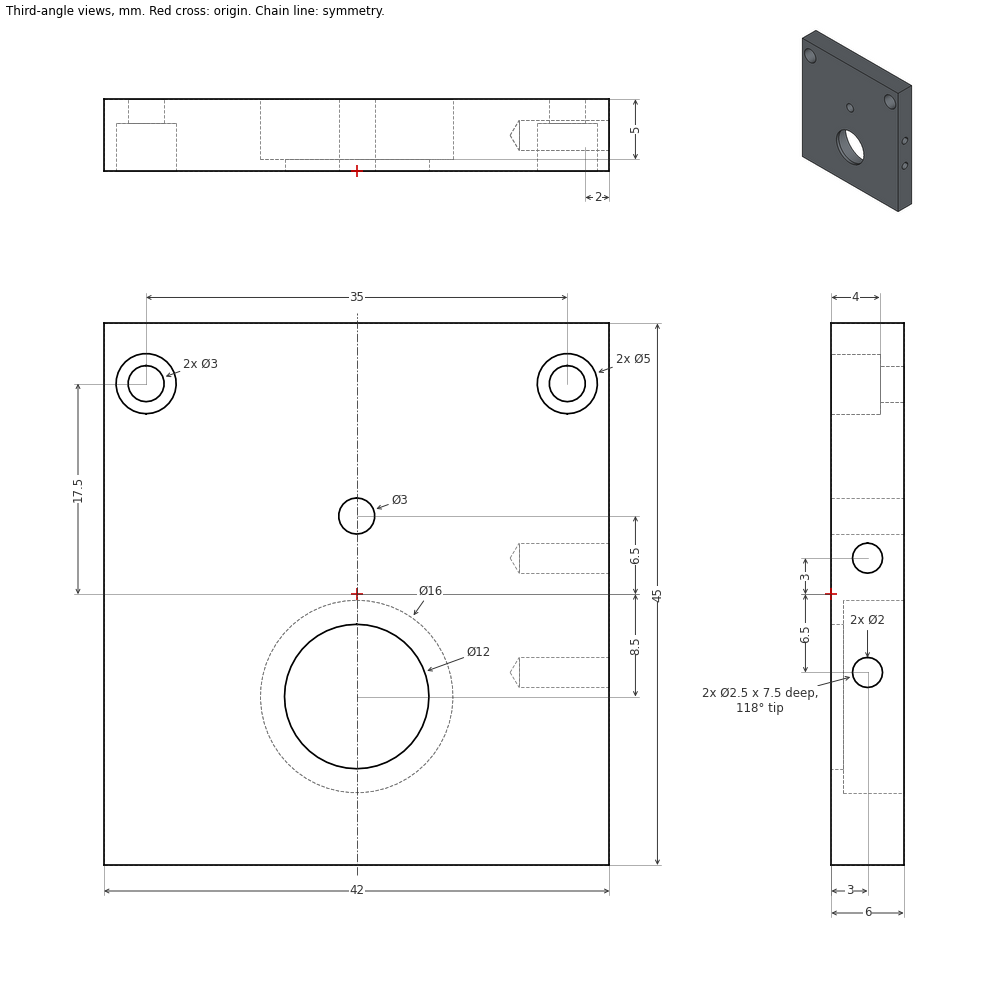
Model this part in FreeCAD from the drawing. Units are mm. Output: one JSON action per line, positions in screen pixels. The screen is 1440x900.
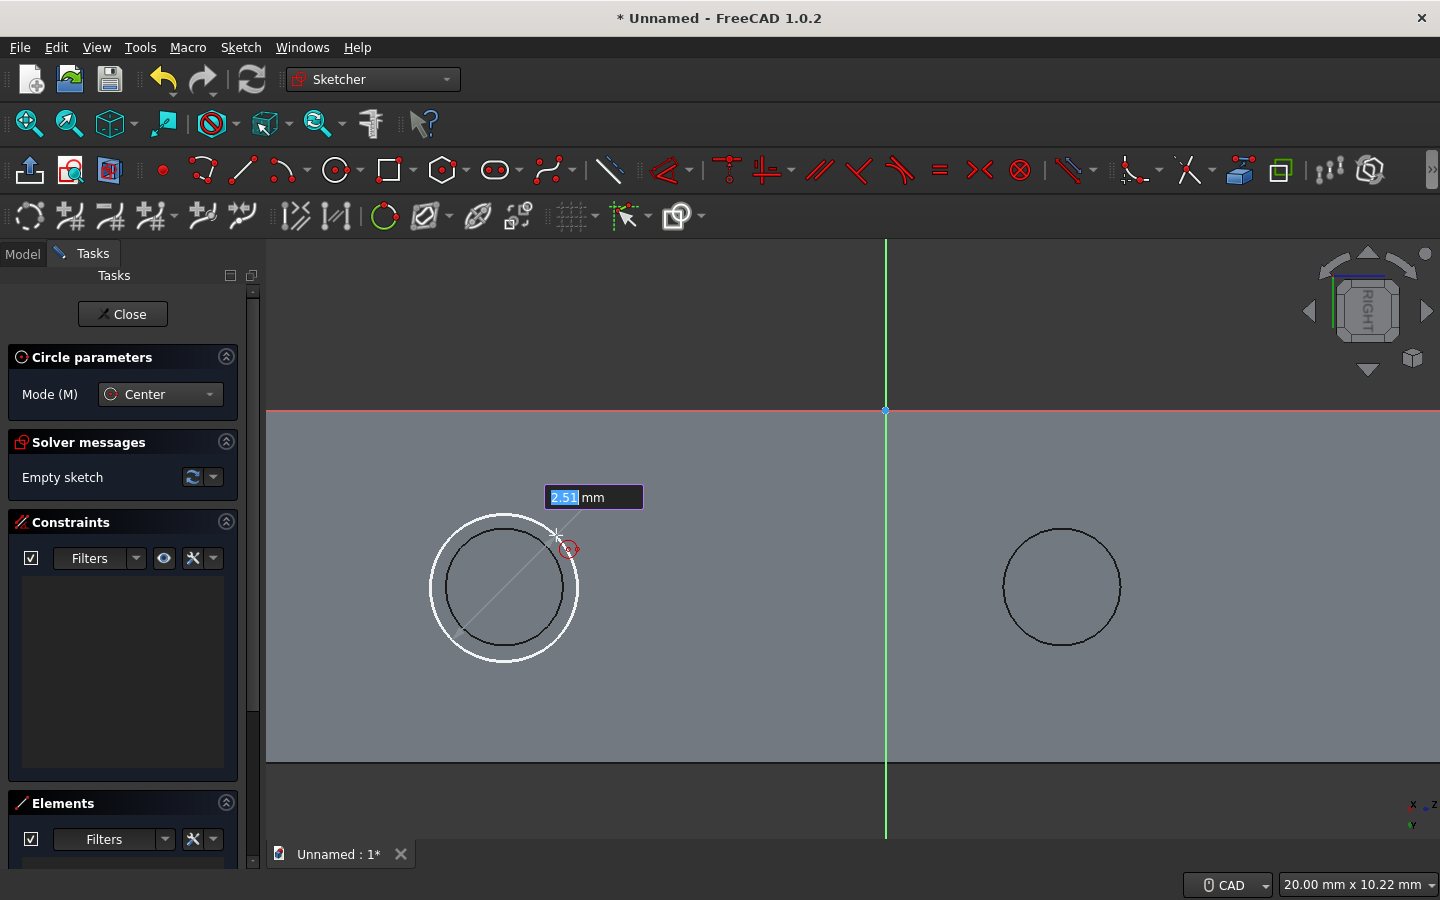
{"action": "type", "text": "2.5"}
{"action": "key", "text": "Return"}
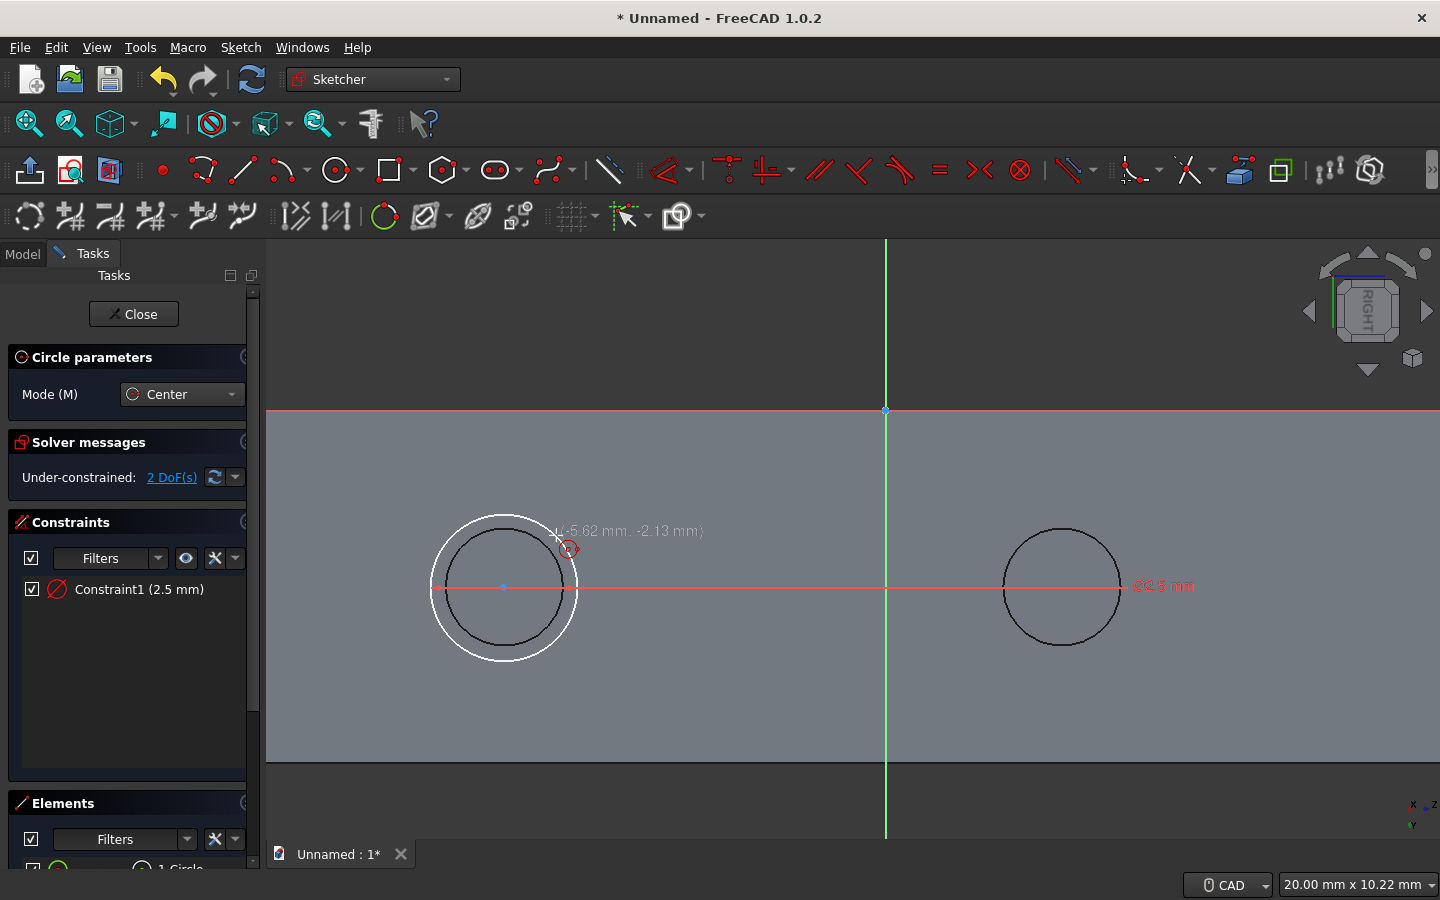
{"action": "left_click", "coordinate": [1062, 587]}
{"action": "mouse_move", "coordinate": [1114, 535]}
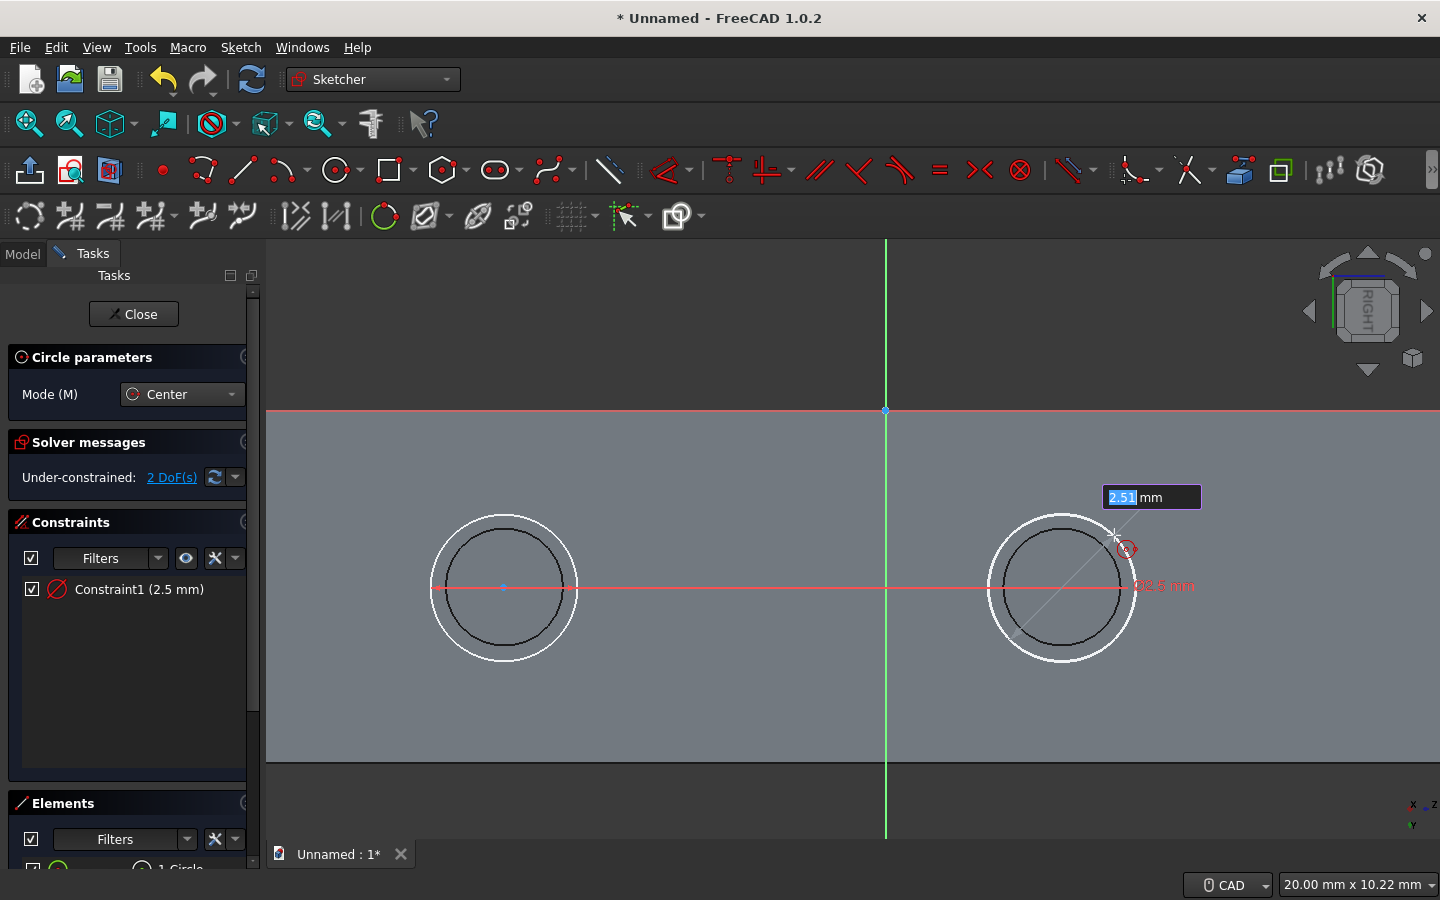
{"action": "type", "text": "2.5"}
{"action": "key", "text": "Return"}
{"action": "key", "text": "Escape"}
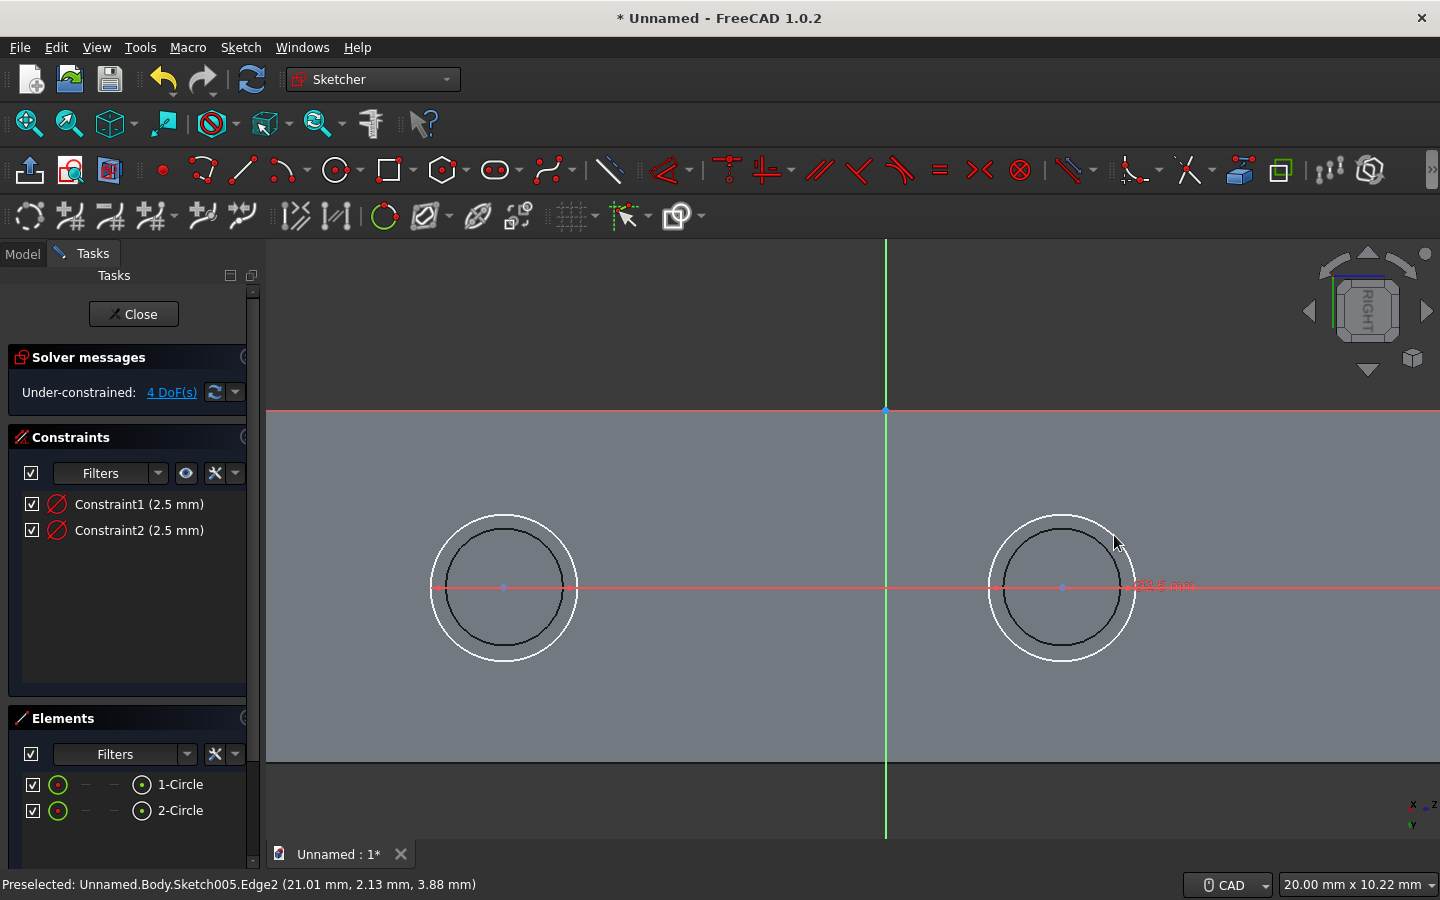
{"action": "key", "text": "d"}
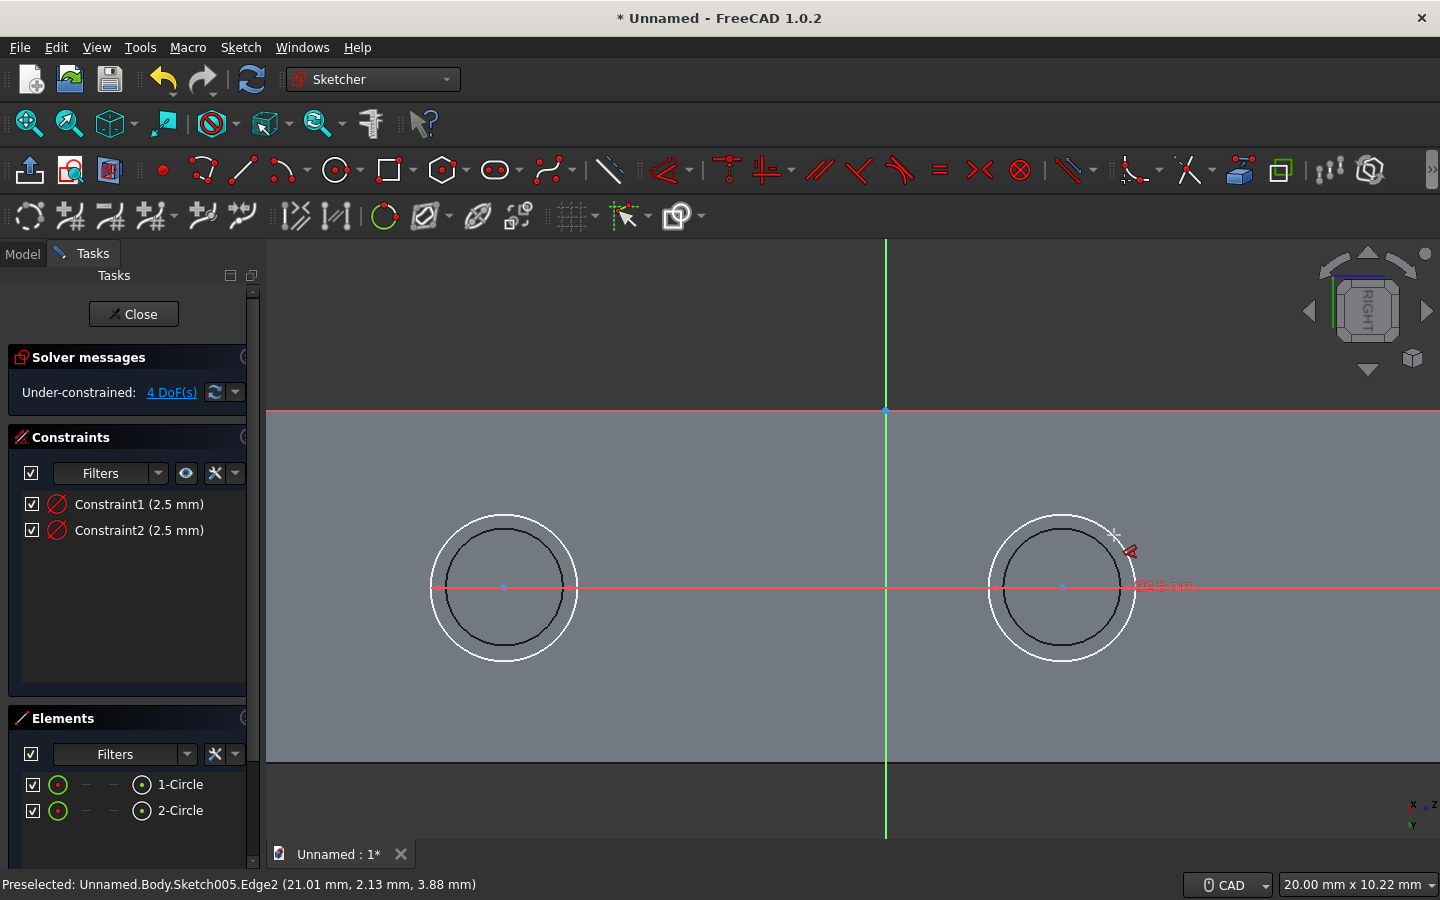
{"action": "left_click", "coordinate": [504, 588]}
{"action": "left_click", "coordinate": [470, 499]}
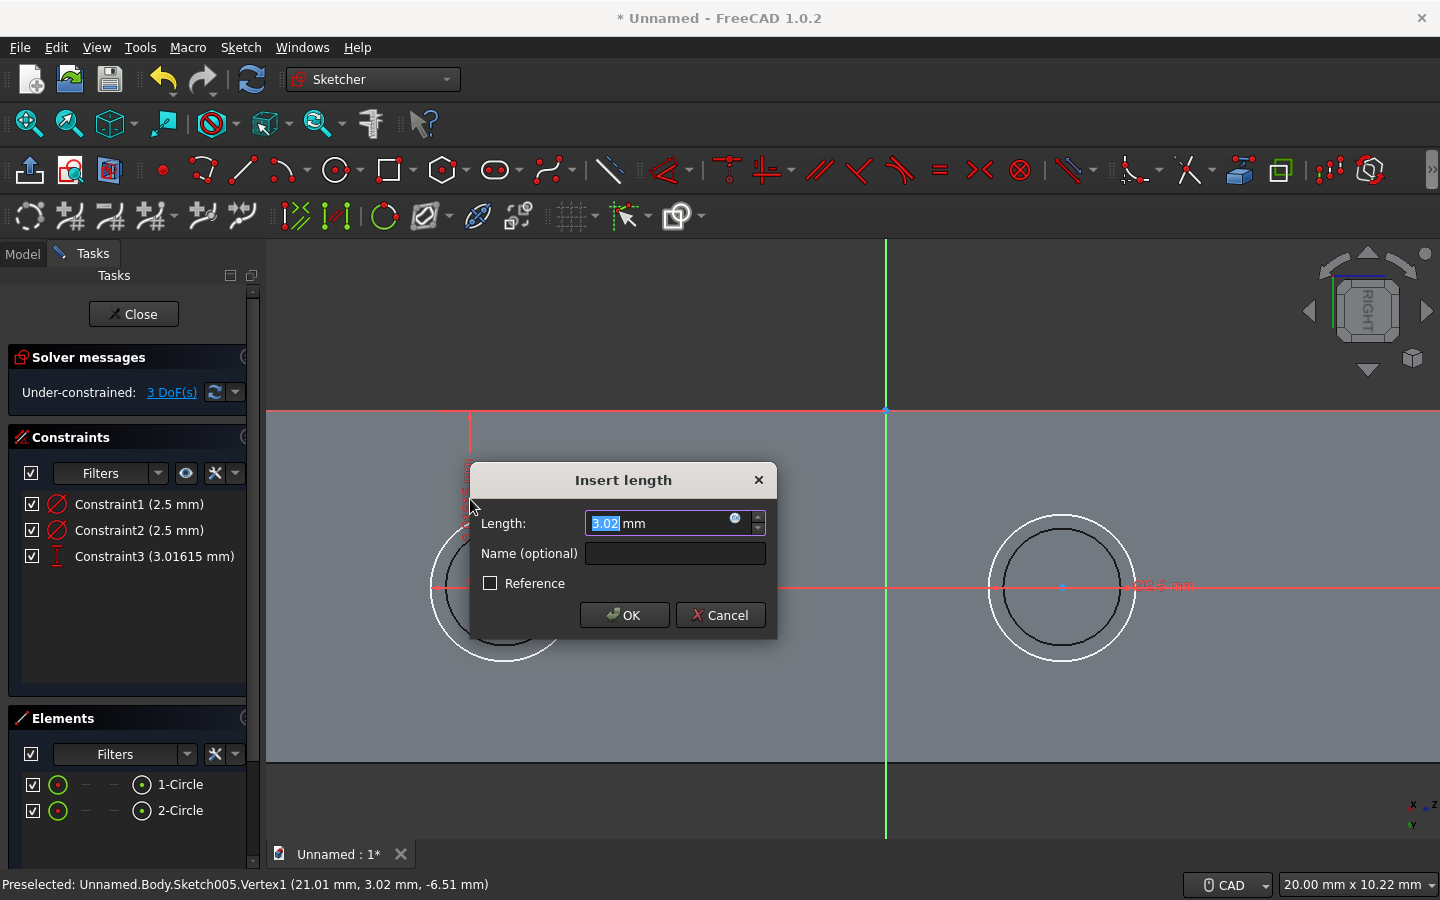
{"action": "type", "text": "3"}
{"action": "key", "text": "Return"}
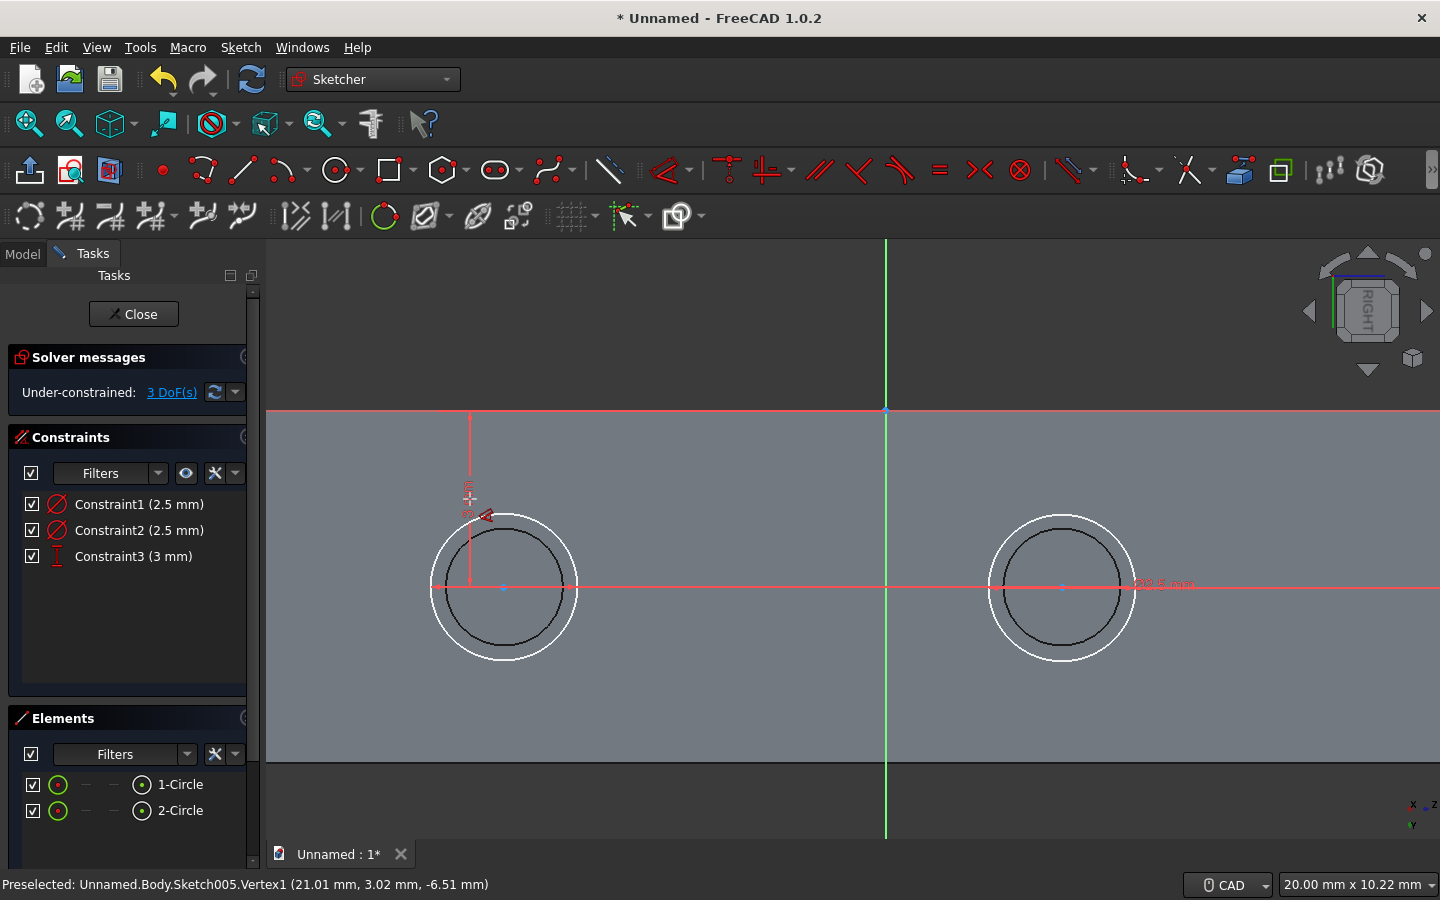
{"action": "left_click", "coordinate": [1062, 588]}
{"action": "left_click", "coordinate": [974, 377]}